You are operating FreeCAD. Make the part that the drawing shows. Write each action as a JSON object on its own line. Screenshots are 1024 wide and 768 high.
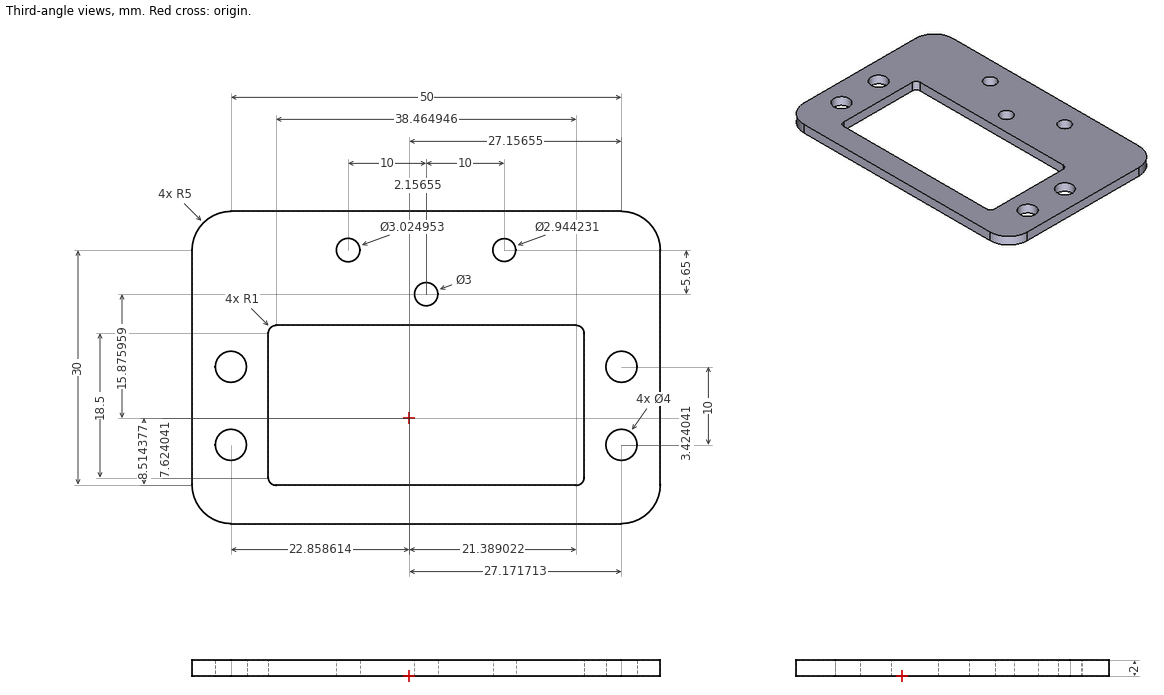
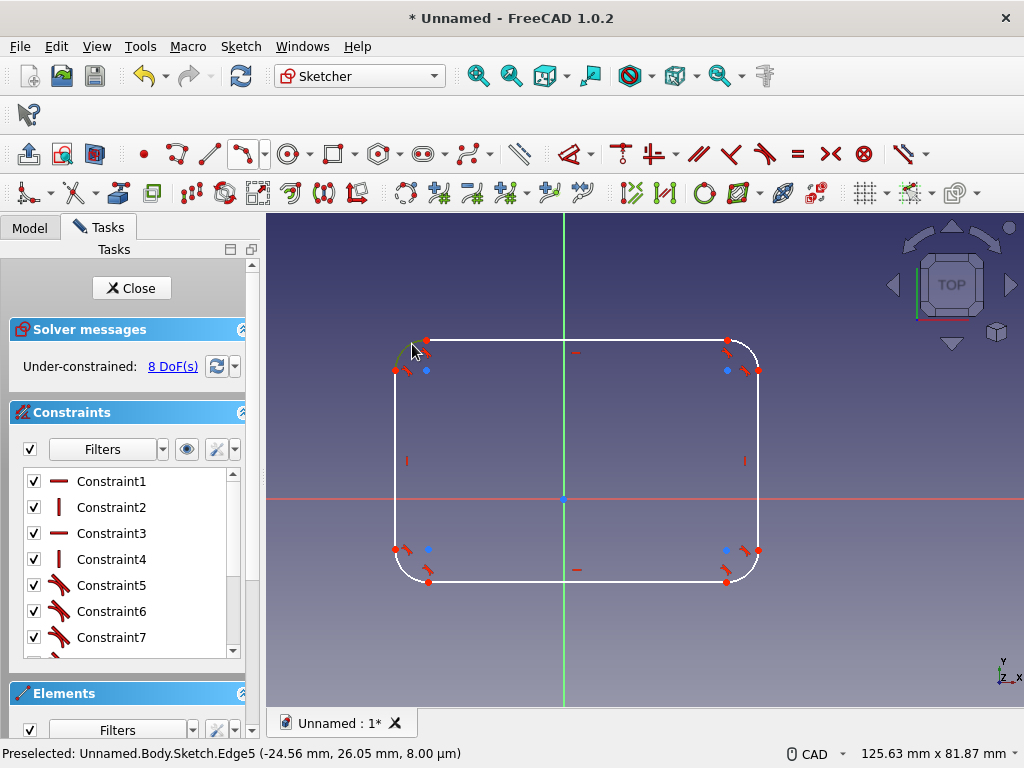
{"action": "left_click", "coordinate": [399, 564]}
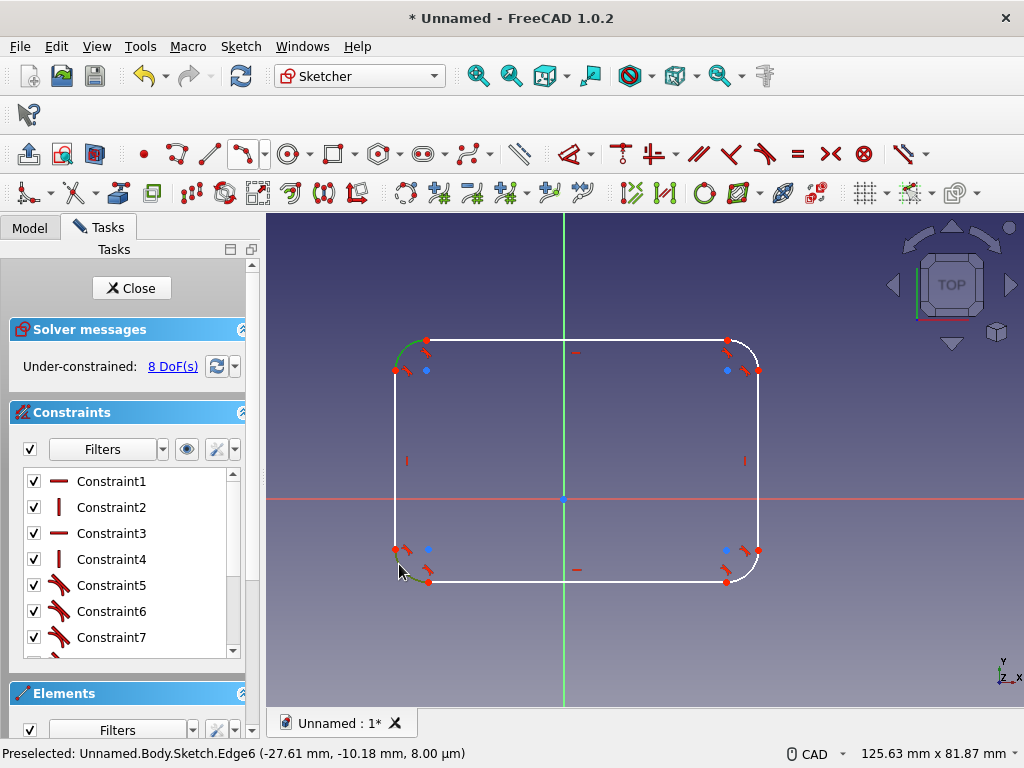
{"action": "left_click", "coordinate": [741, 579]}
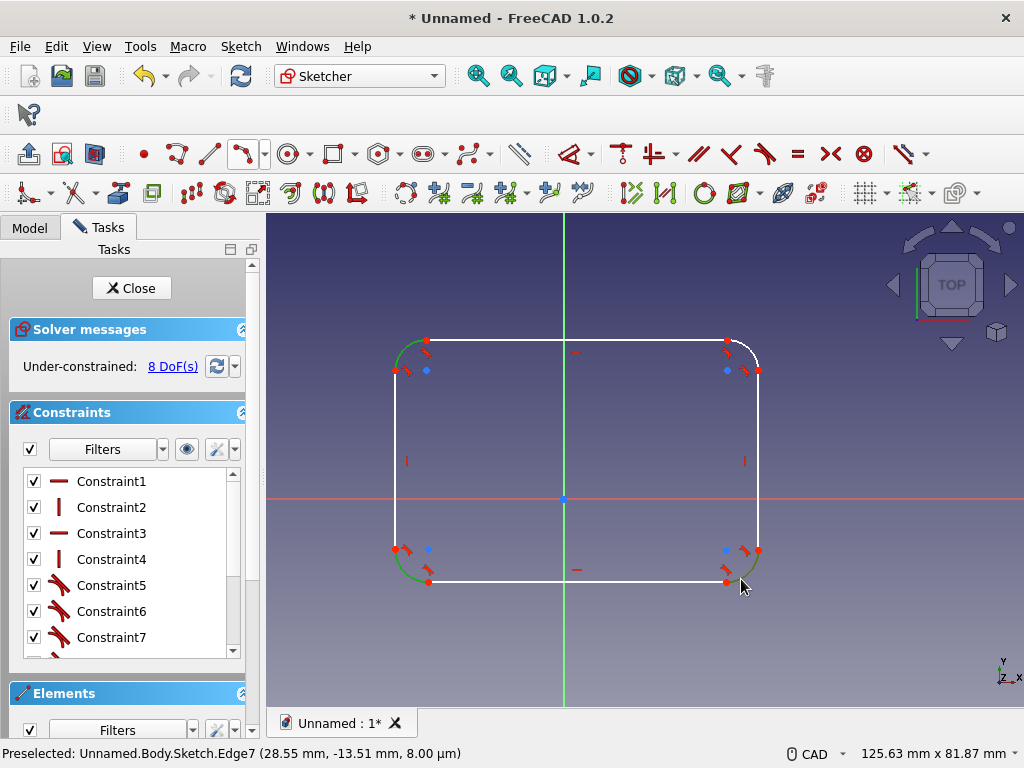
{"action": "left_click", "coordinate": [755, 357]}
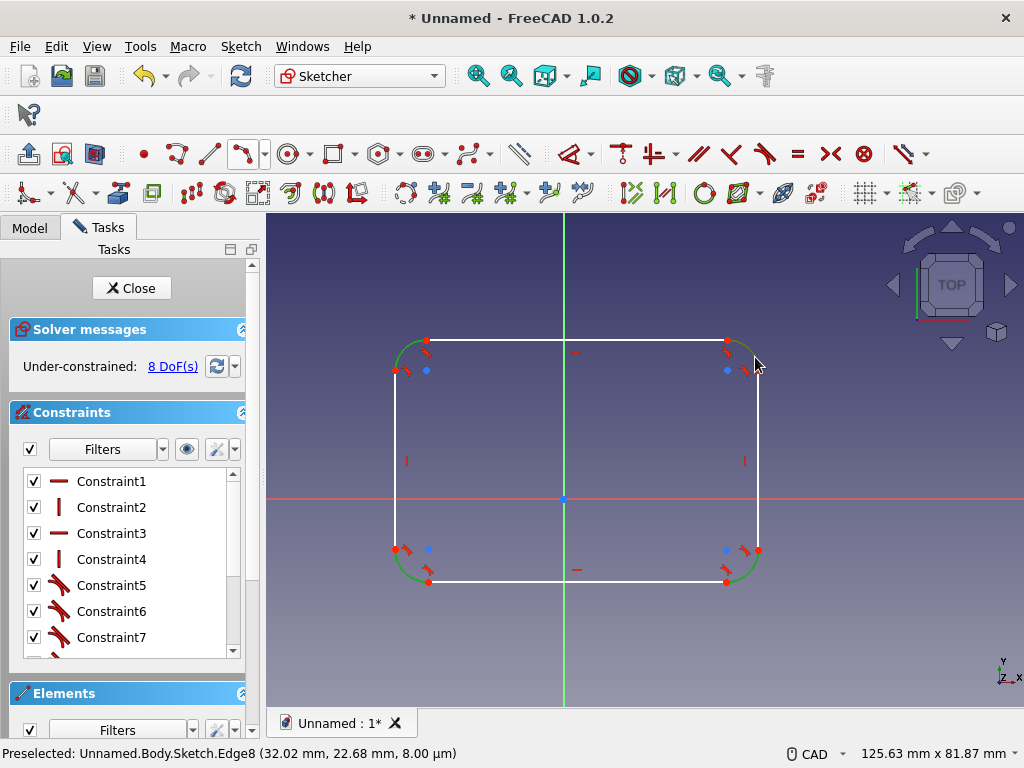
{"action": "left_click", "coordinate": [798, 154]}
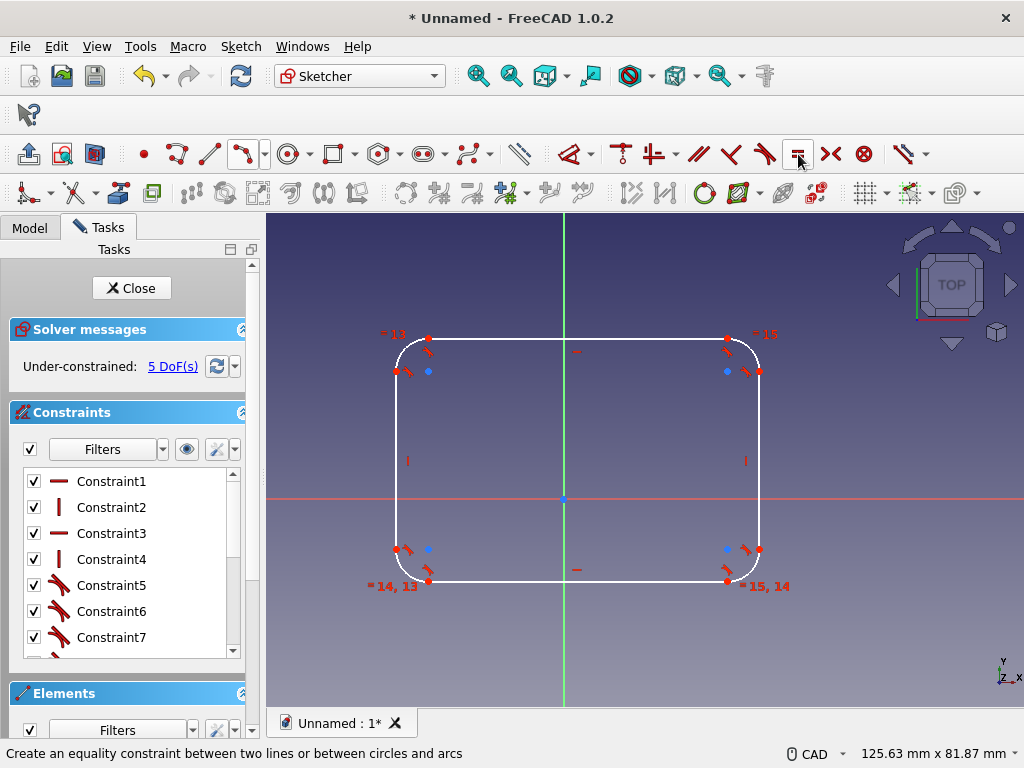
{"action": "left_click", "coordinate": [568, 154]}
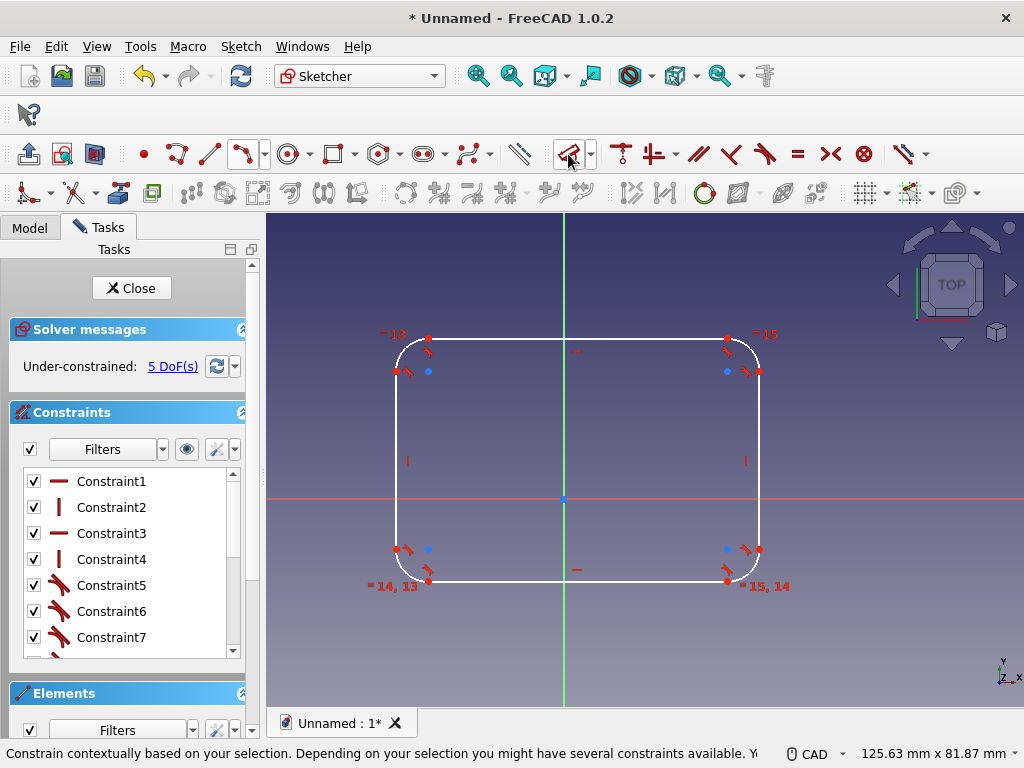
{"action": "scroll", "coordinate": [414, 342], "scroll_direction": "up", "scroll_amount": 2}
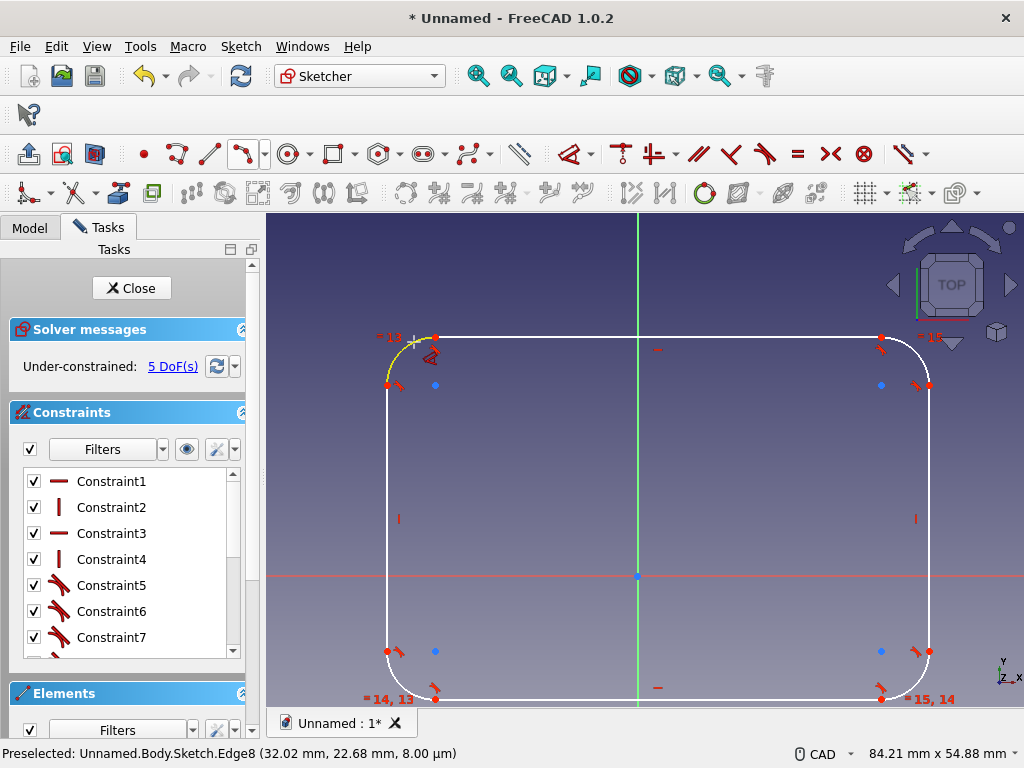
{"action": "left_click", "coordinate": [413, 343]}
{"action": "left_click", "coordinate": [398, 315]}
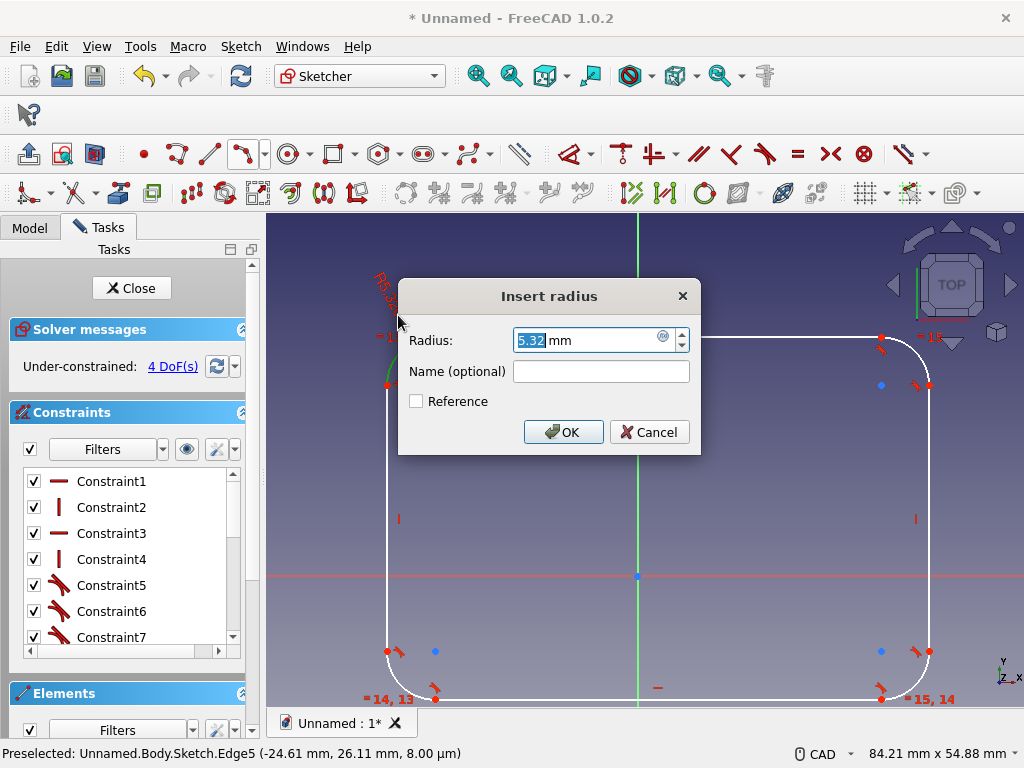
{"action": "type", "text": "5"}
{"action": "key", "text": "Return"}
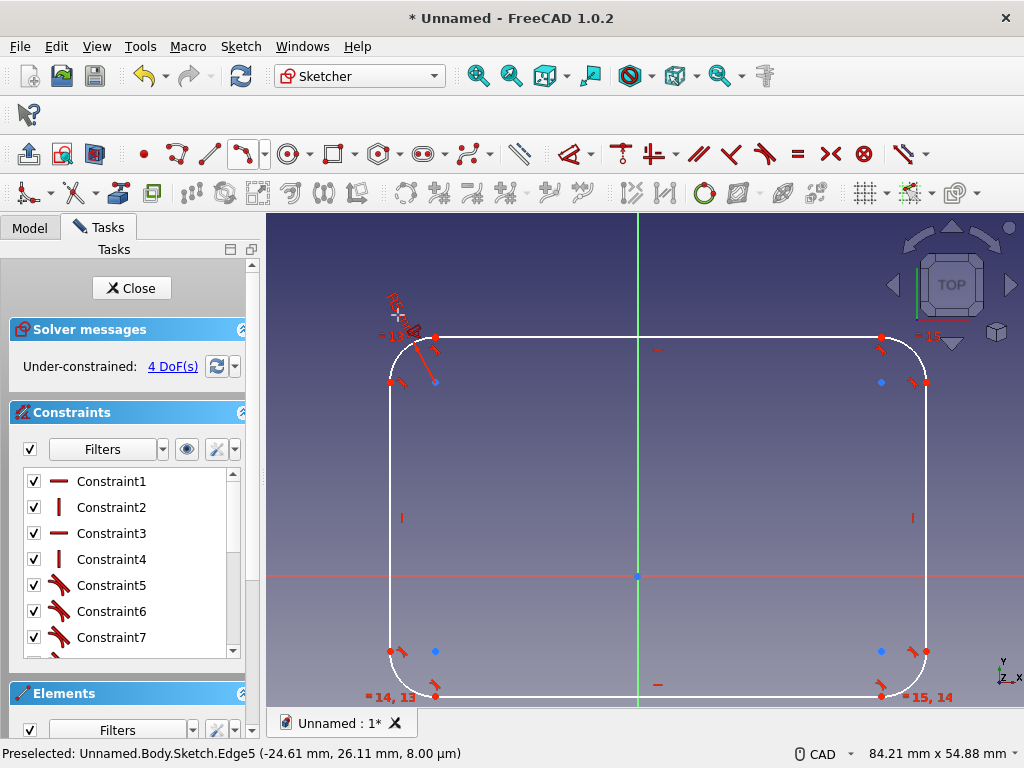
{"action": "left_click", "coordinate": [747, 337]}
{"action": "left_click", "coordinate": [550, 303]}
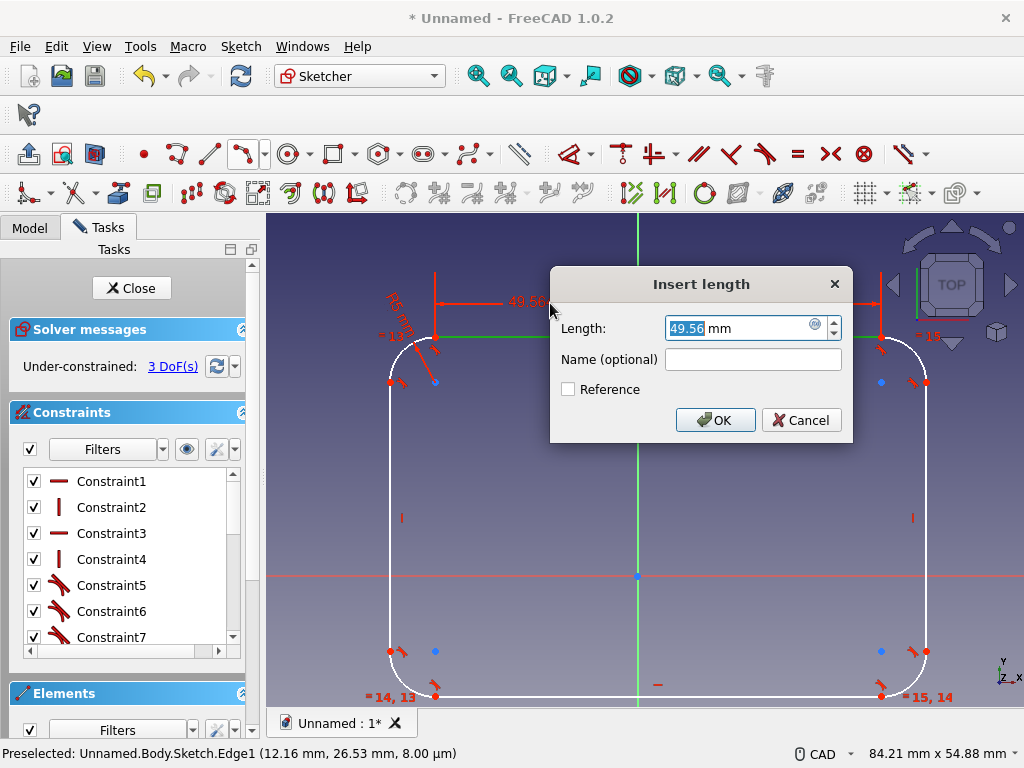
{"action": "type", "text": "50"}
{"action": "key", "text": "Return"}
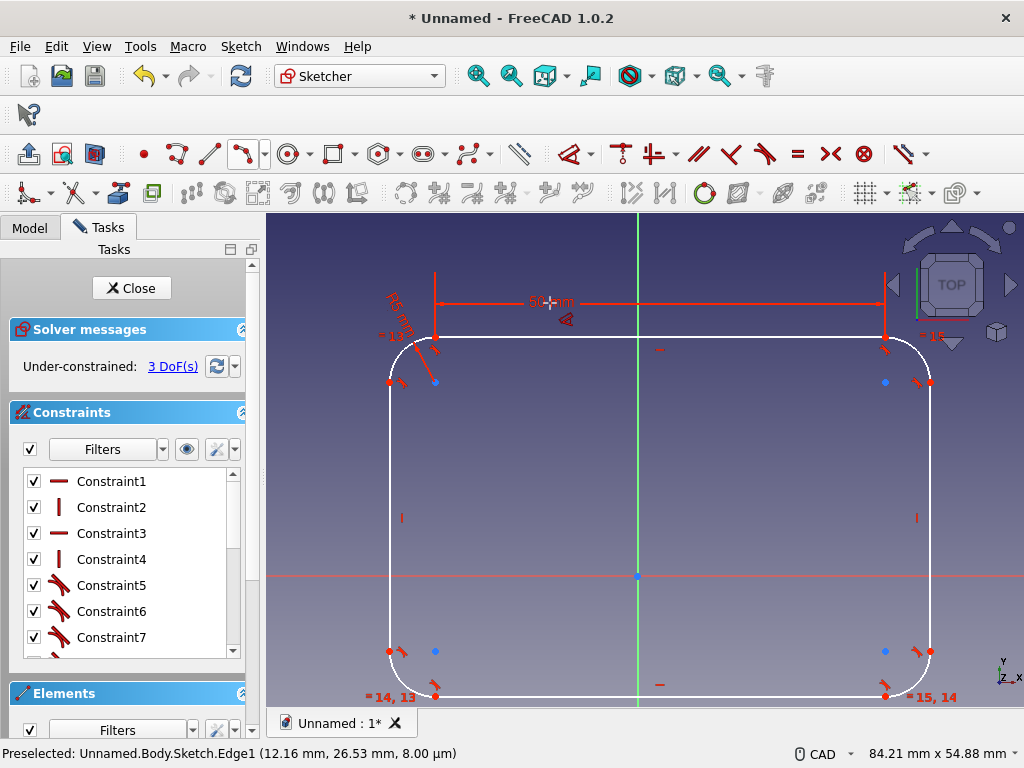
{"action": "left_click", "coordinate": [390, 463]}
{"action": "left_click", "coordinate": [356, 517]}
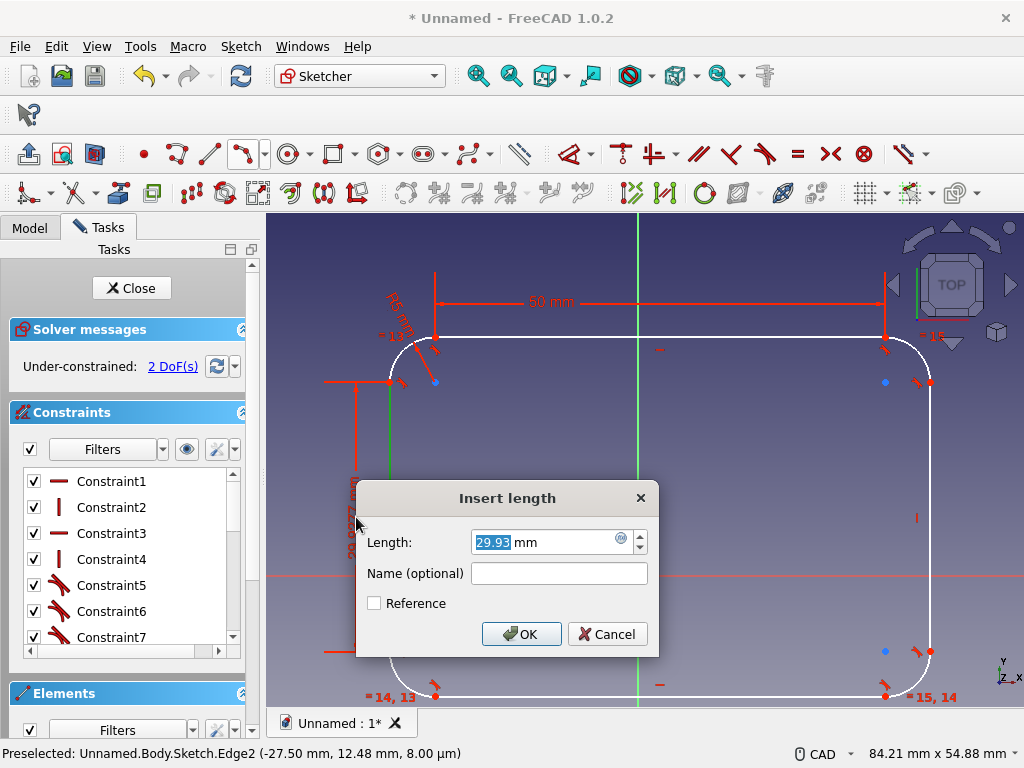
{"action": "type", "text": "30"}
{"action": "key", "text": "Return"}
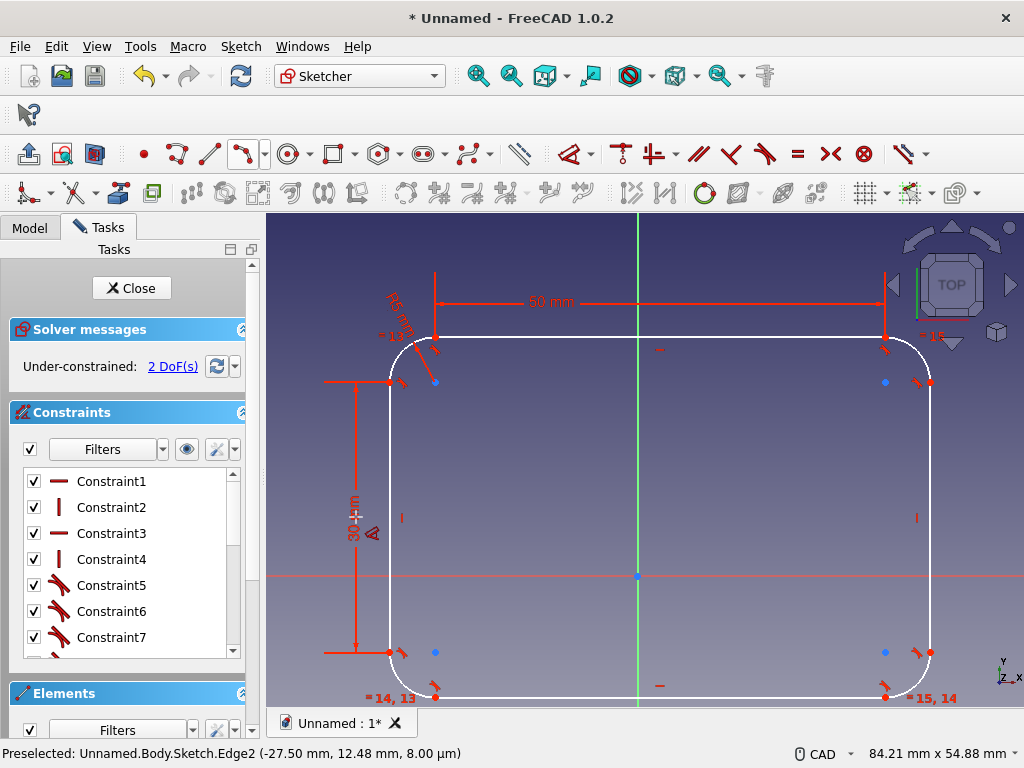
{"action": "scroll", "coordinate": [413, 342], "scroll_direction": "down", "scroll_amount": 2}